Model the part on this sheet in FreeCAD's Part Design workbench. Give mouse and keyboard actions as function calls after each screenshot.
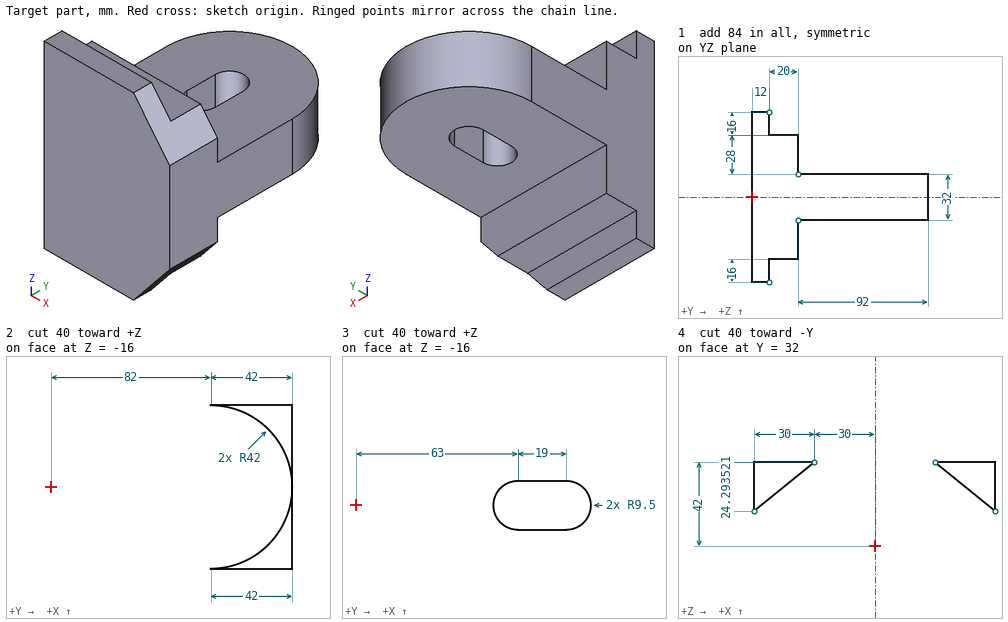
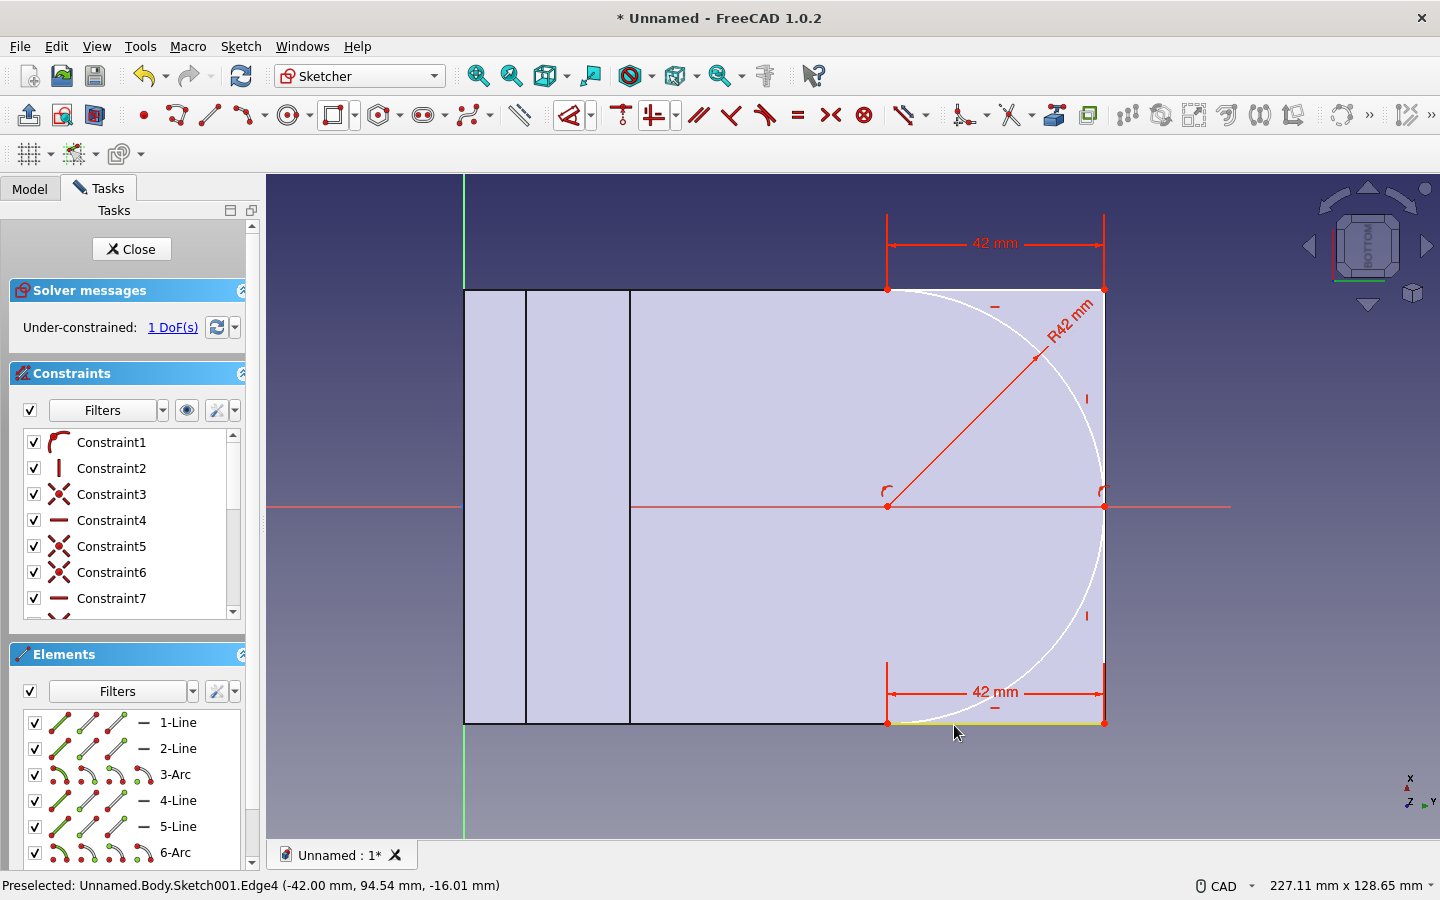
click(887, 290)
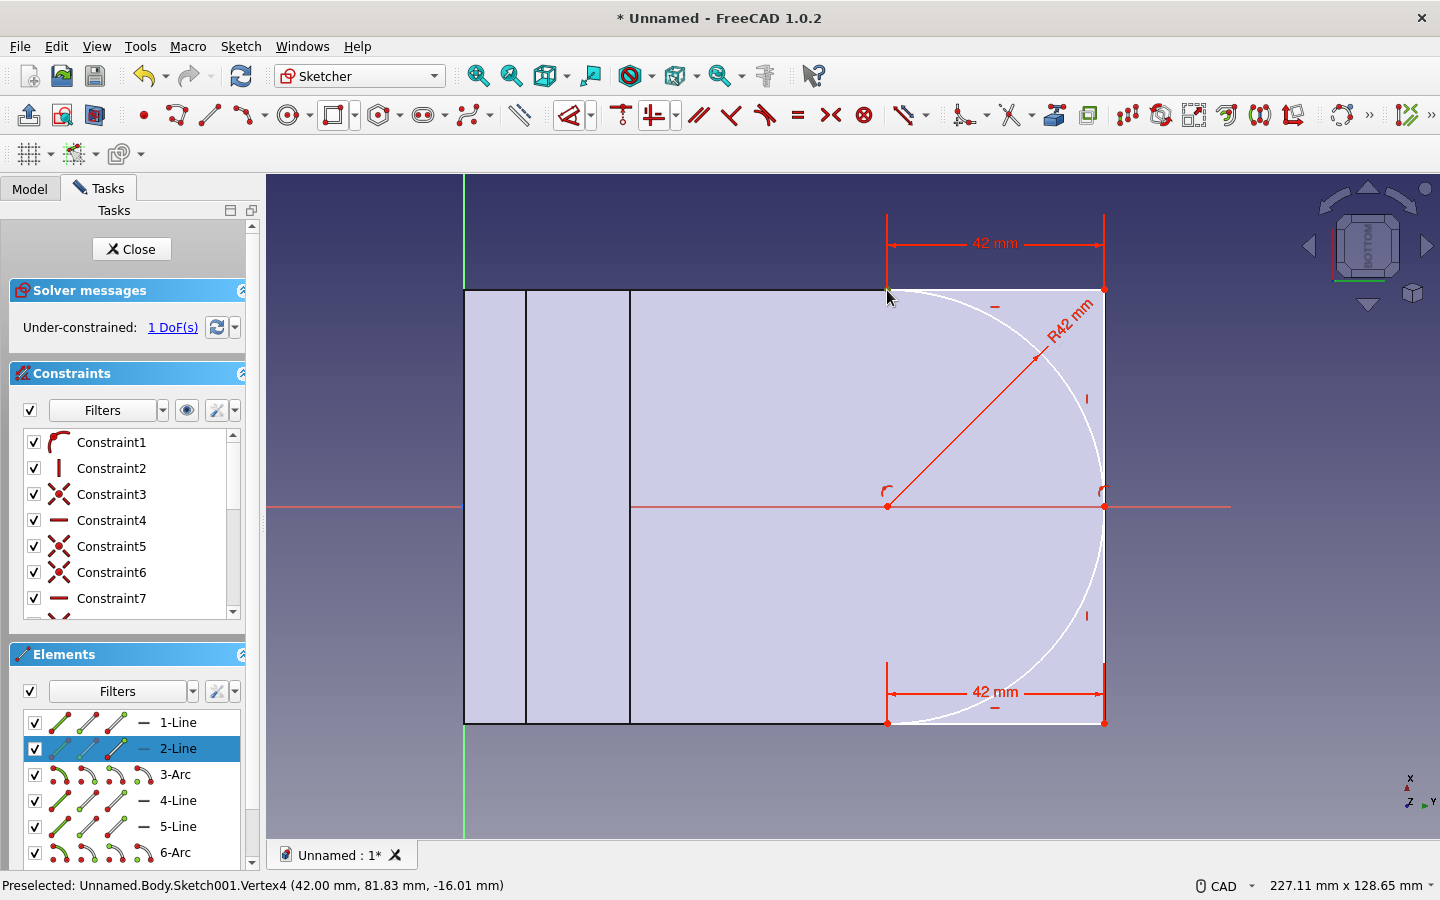
key(l)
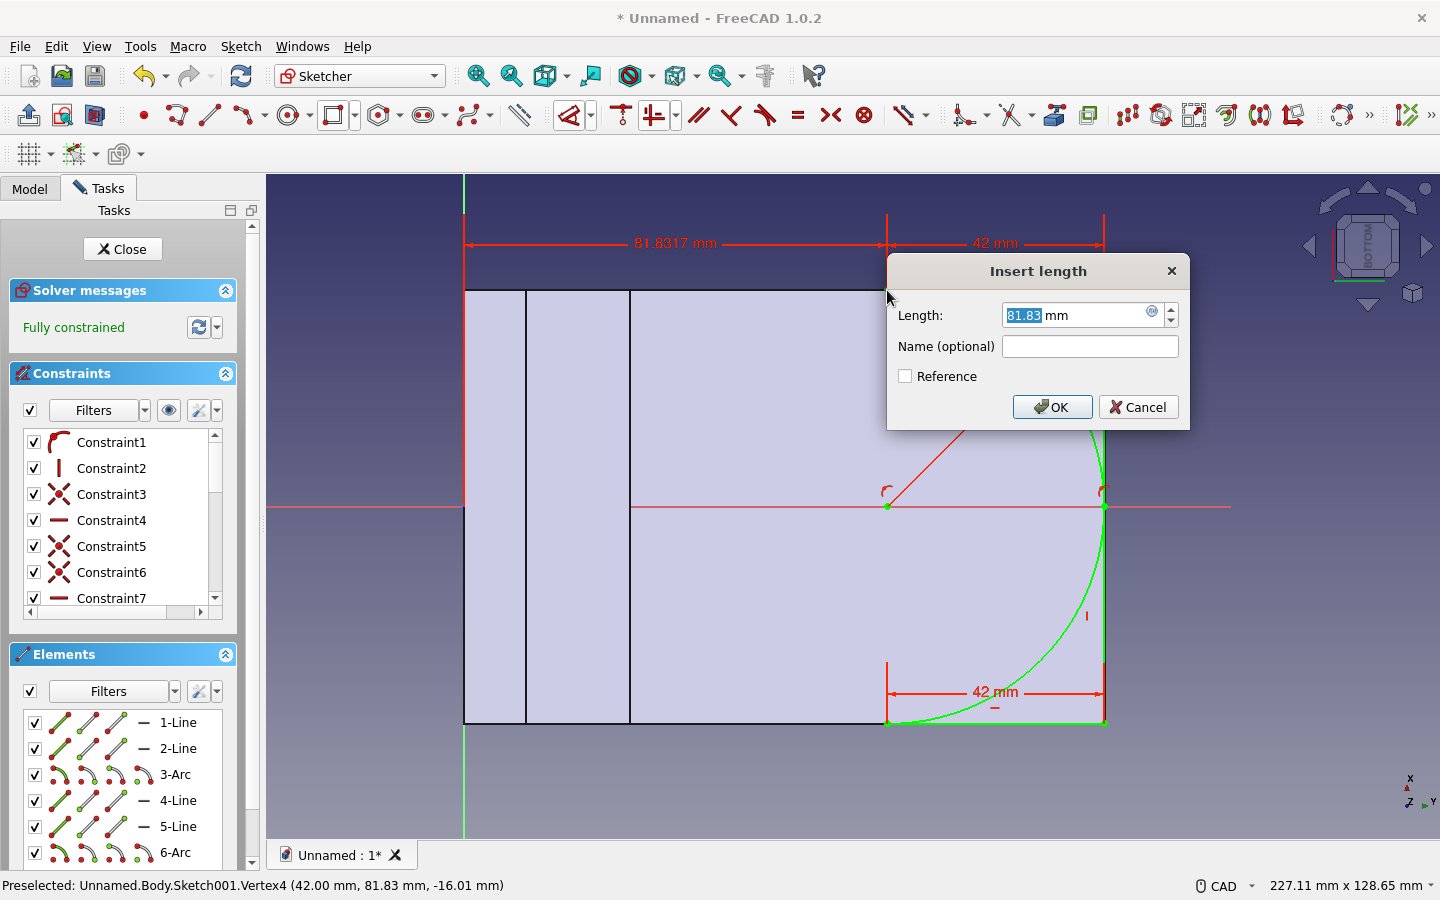
text(82)
key(Return)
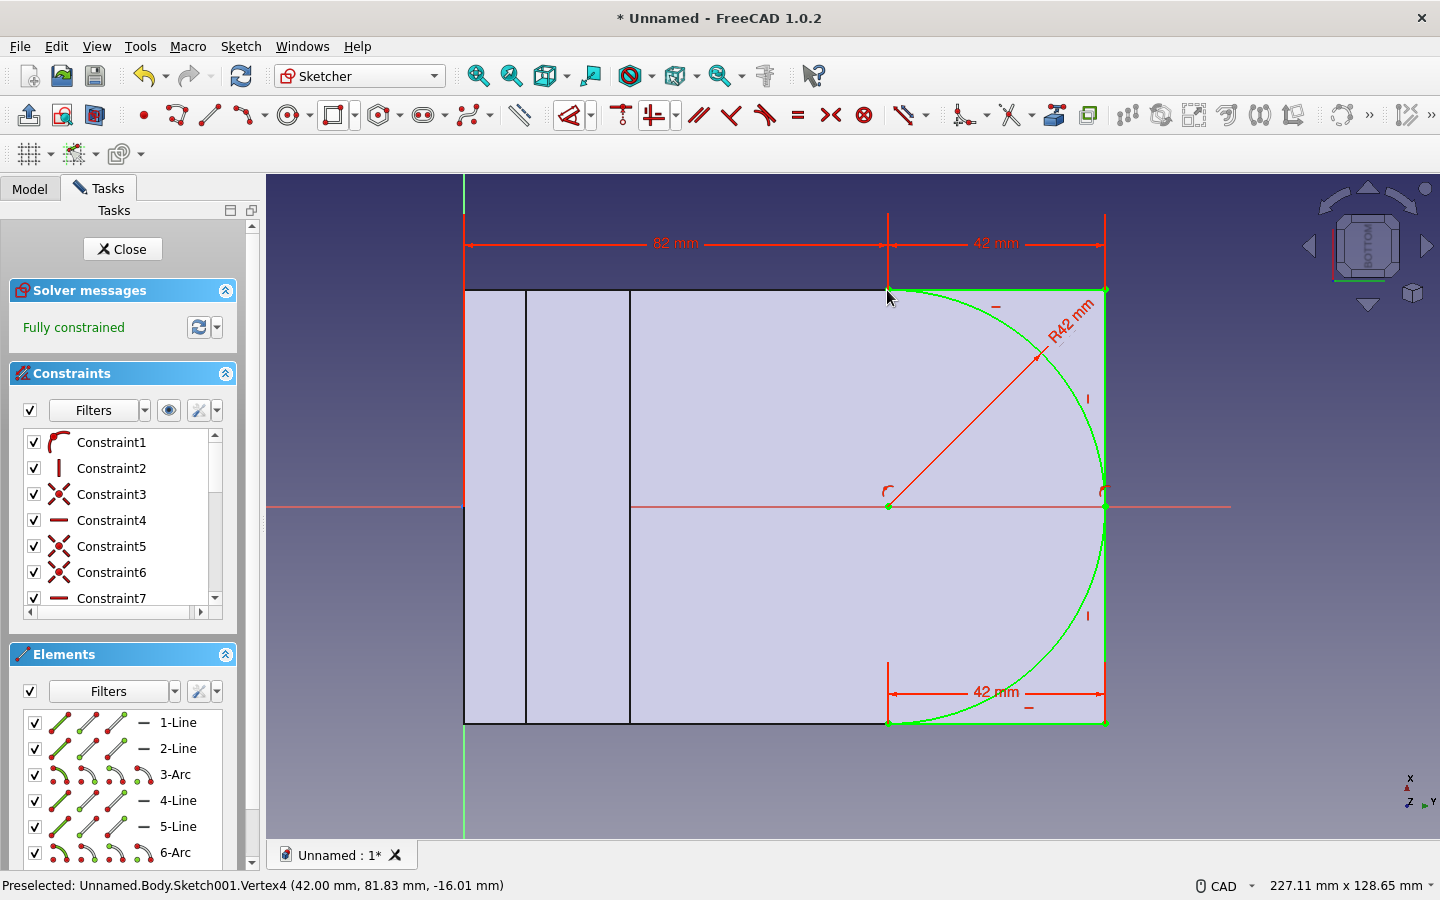
click(123, 249)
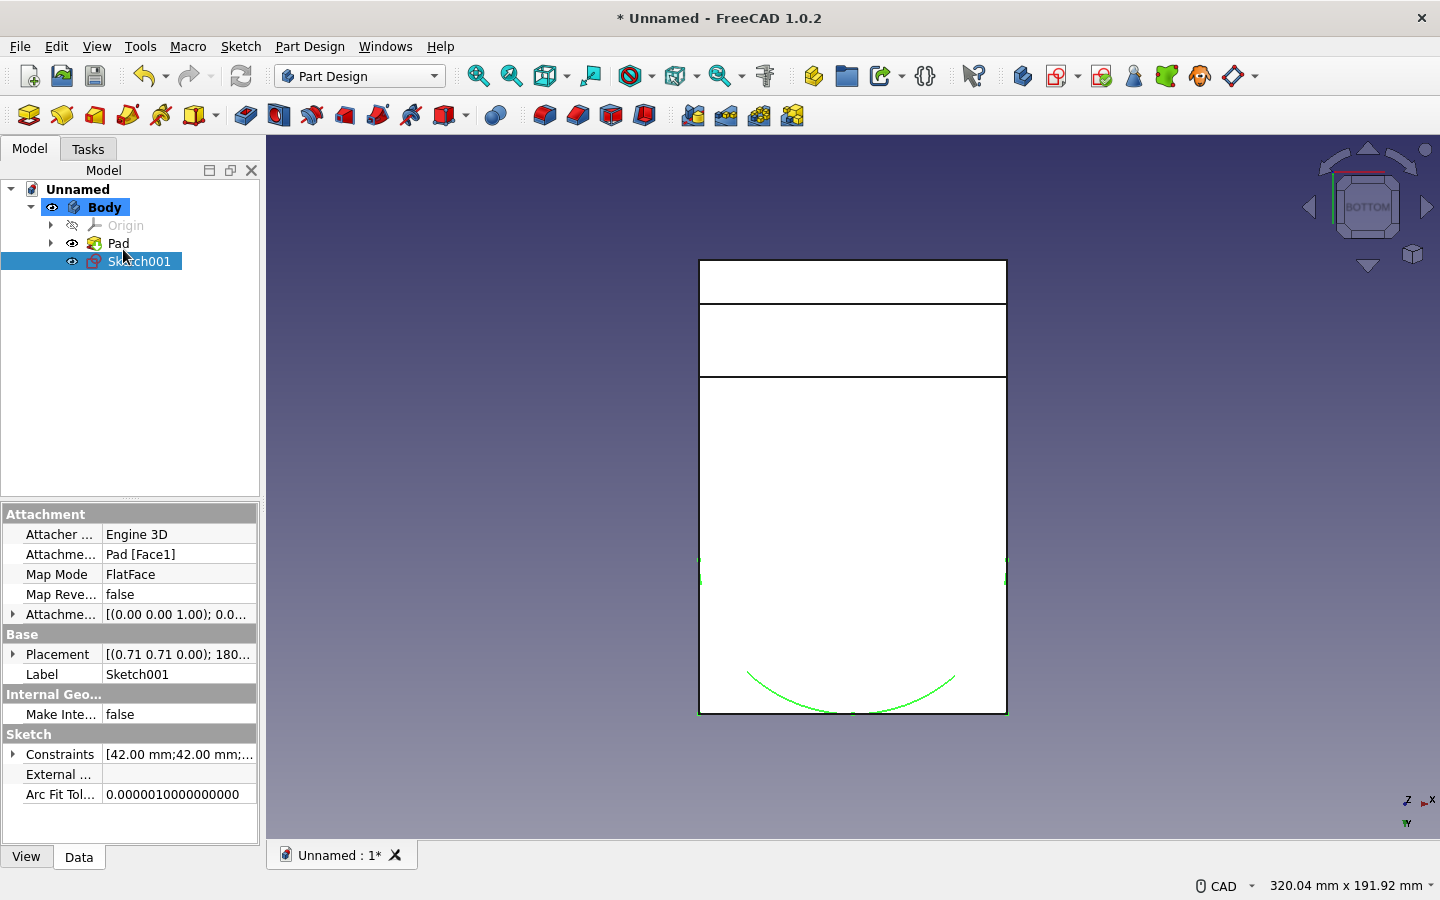
click(246, 116)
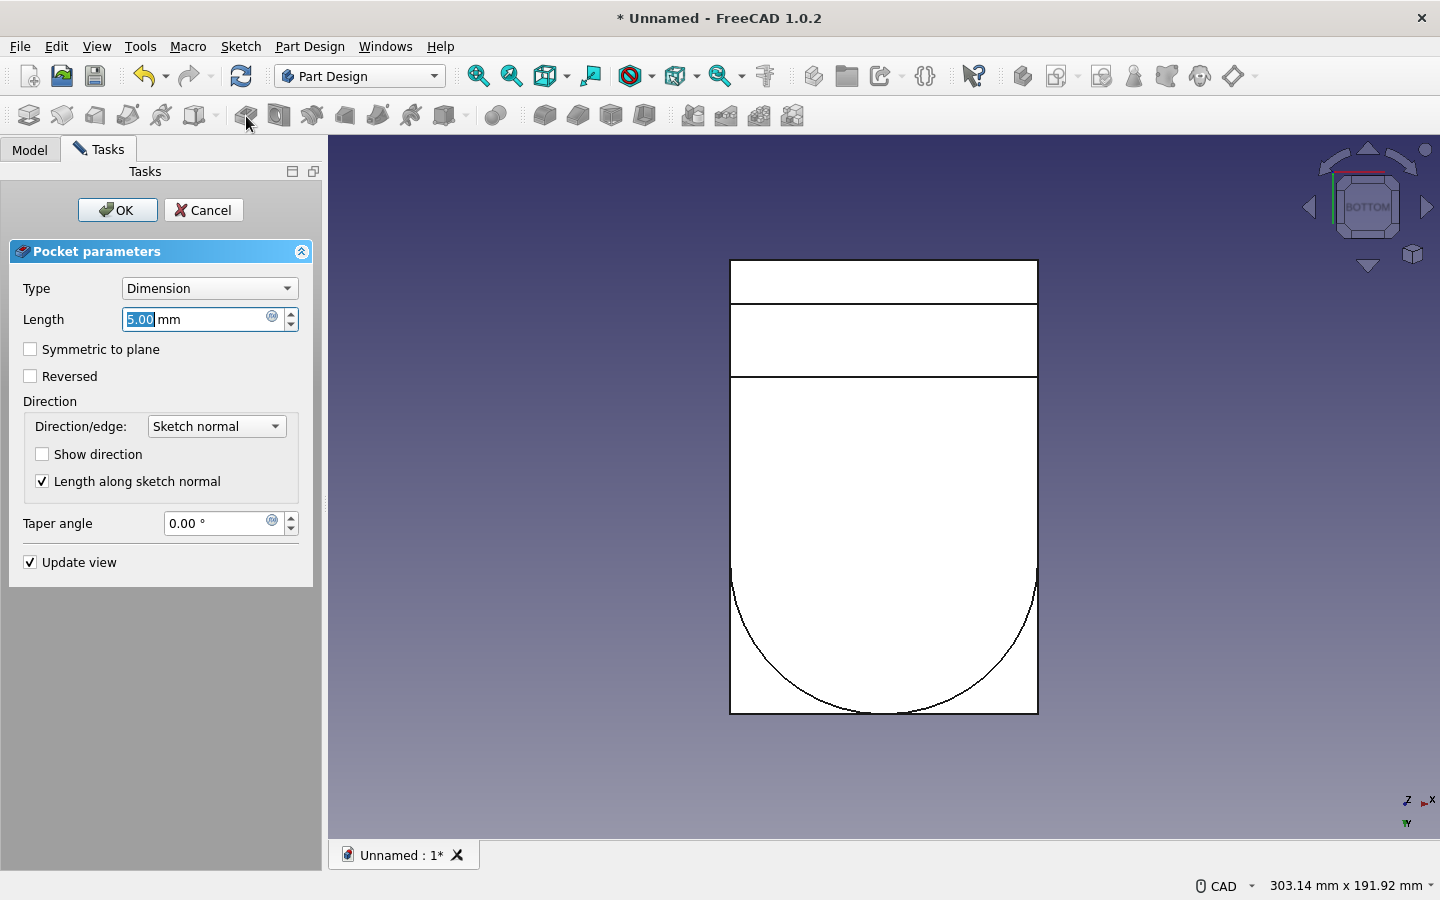
text(40)
key(Tab)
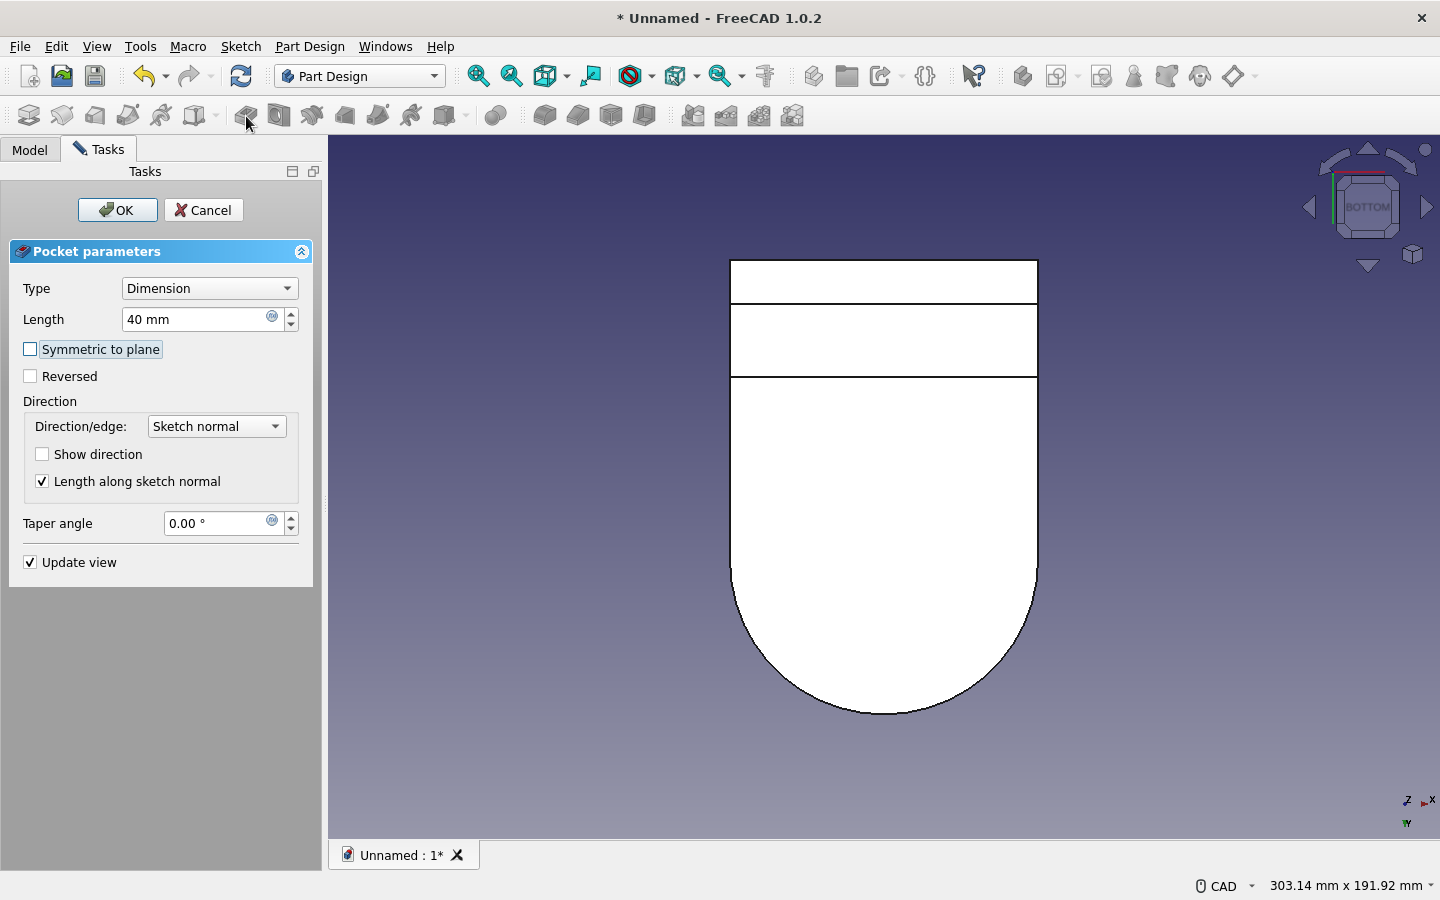
click(118, 210)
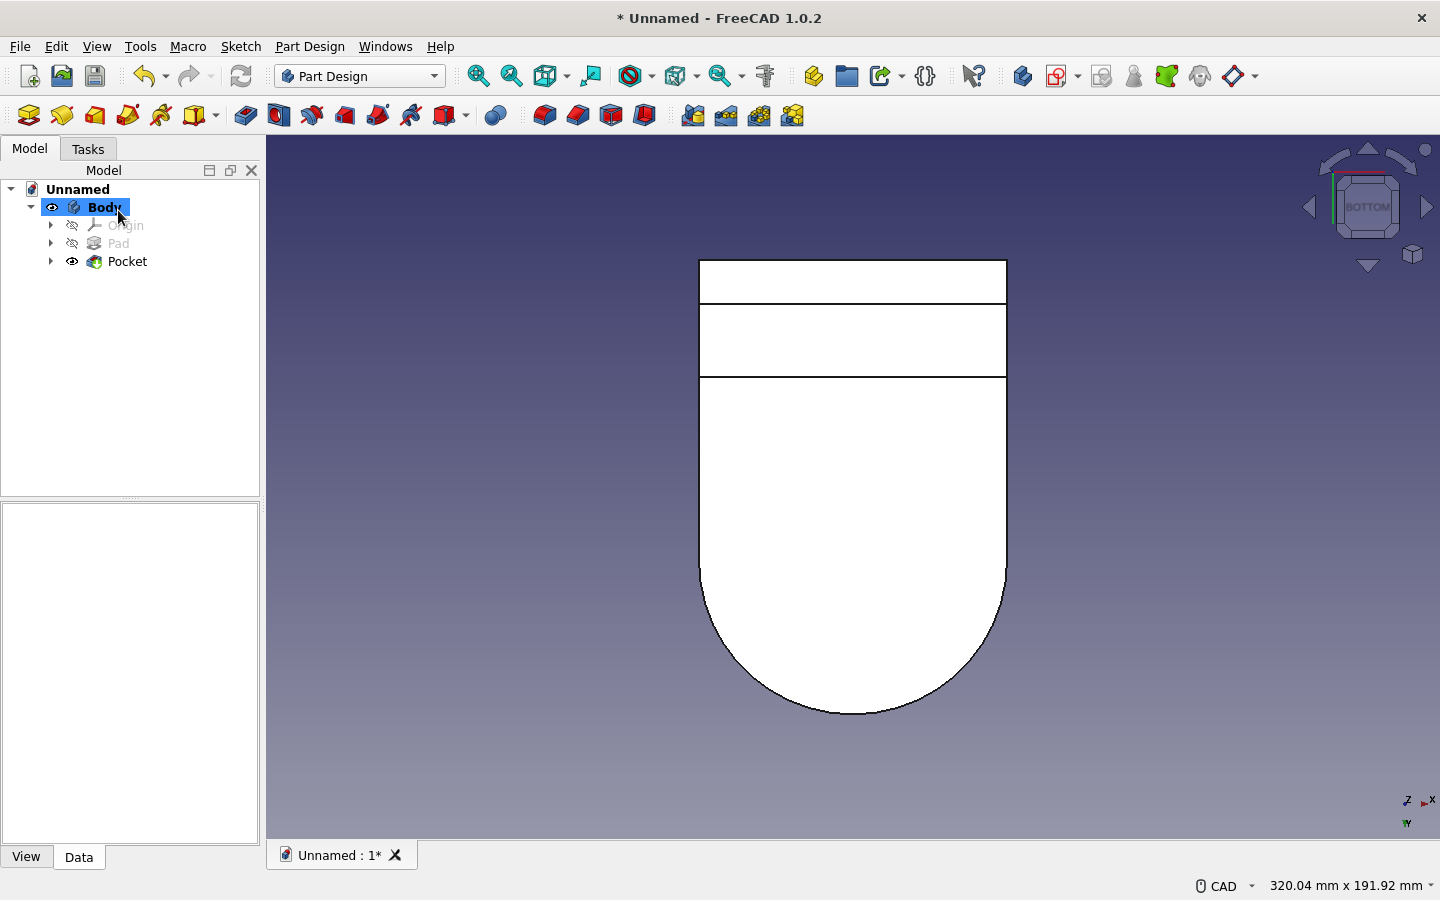
click(853, 545)